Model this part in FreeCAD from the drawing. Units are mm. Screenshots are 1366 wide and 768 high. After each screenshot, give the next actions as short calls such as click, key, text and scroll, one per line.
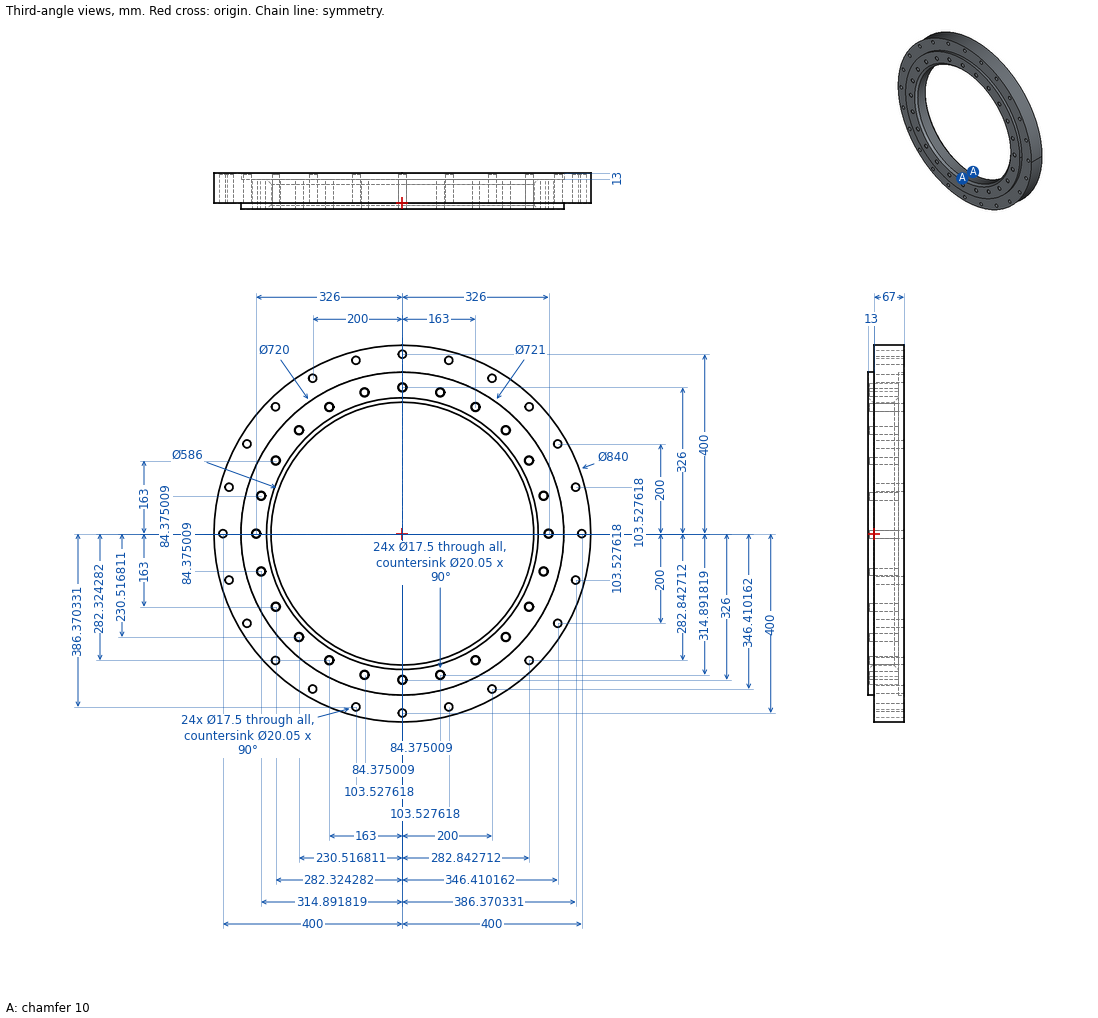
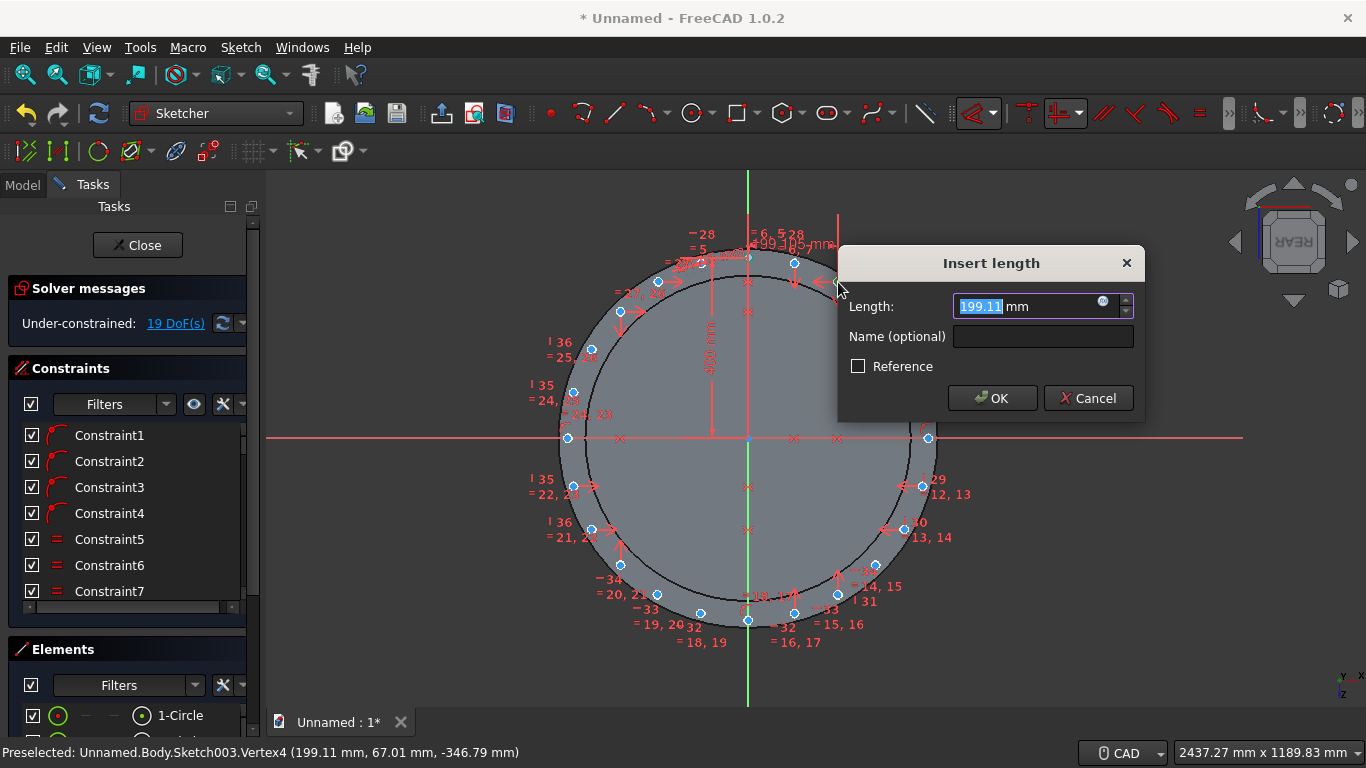
text(200)
key(Return)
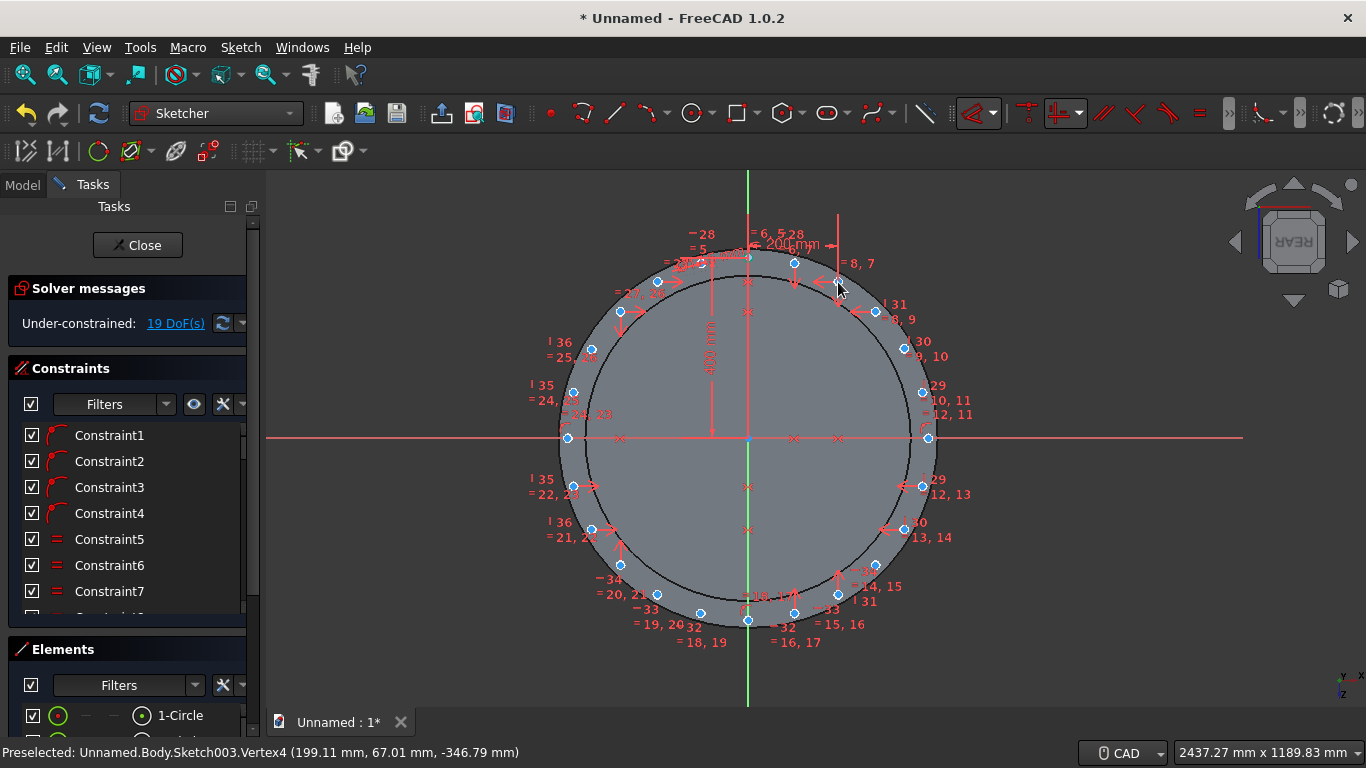
click(904, 349)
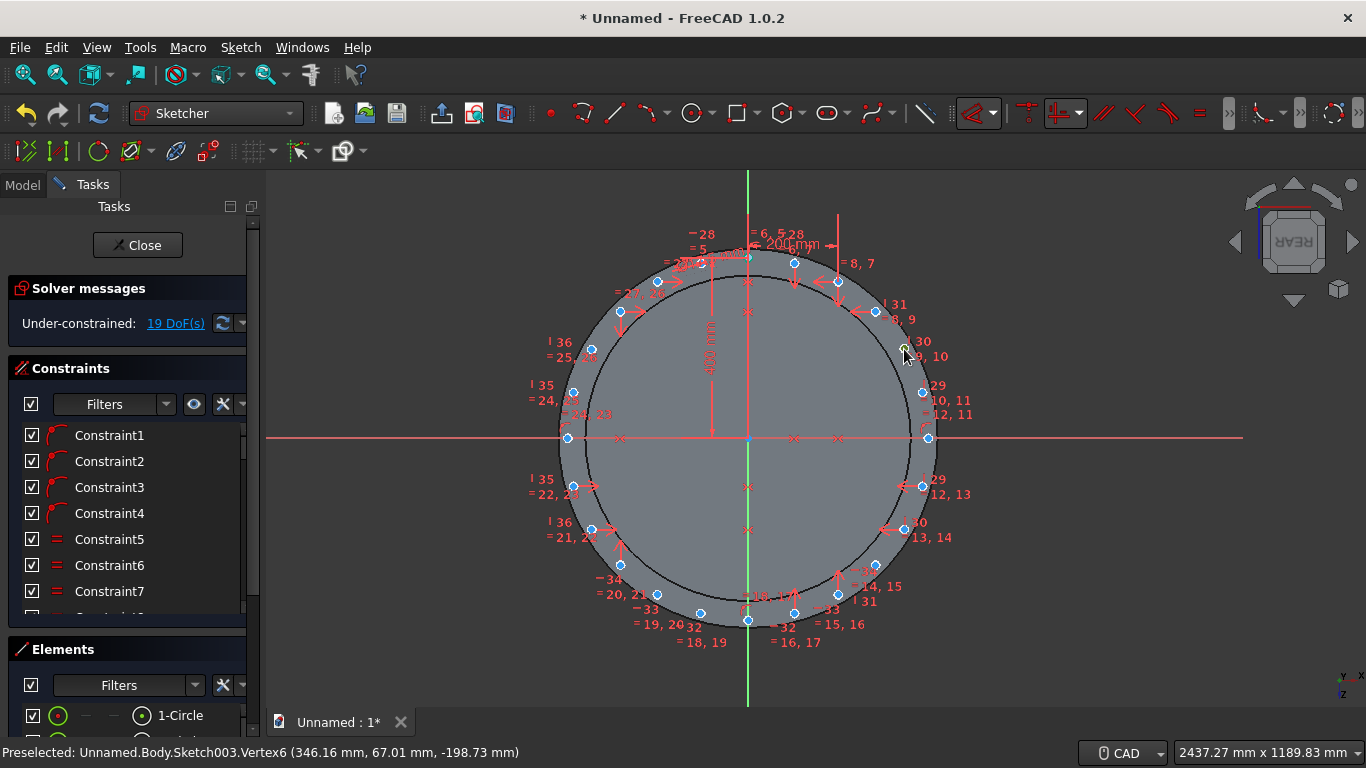
key(i)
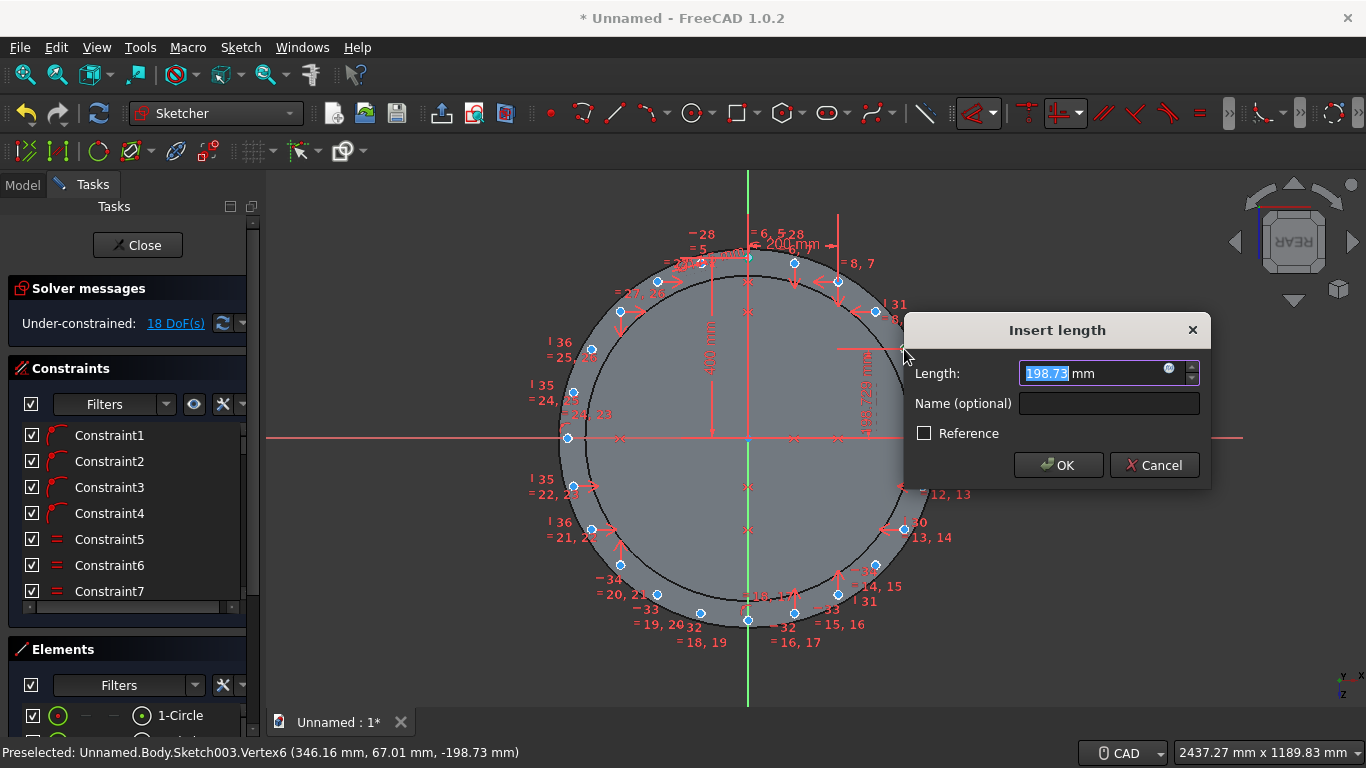
text(200)
key(Return)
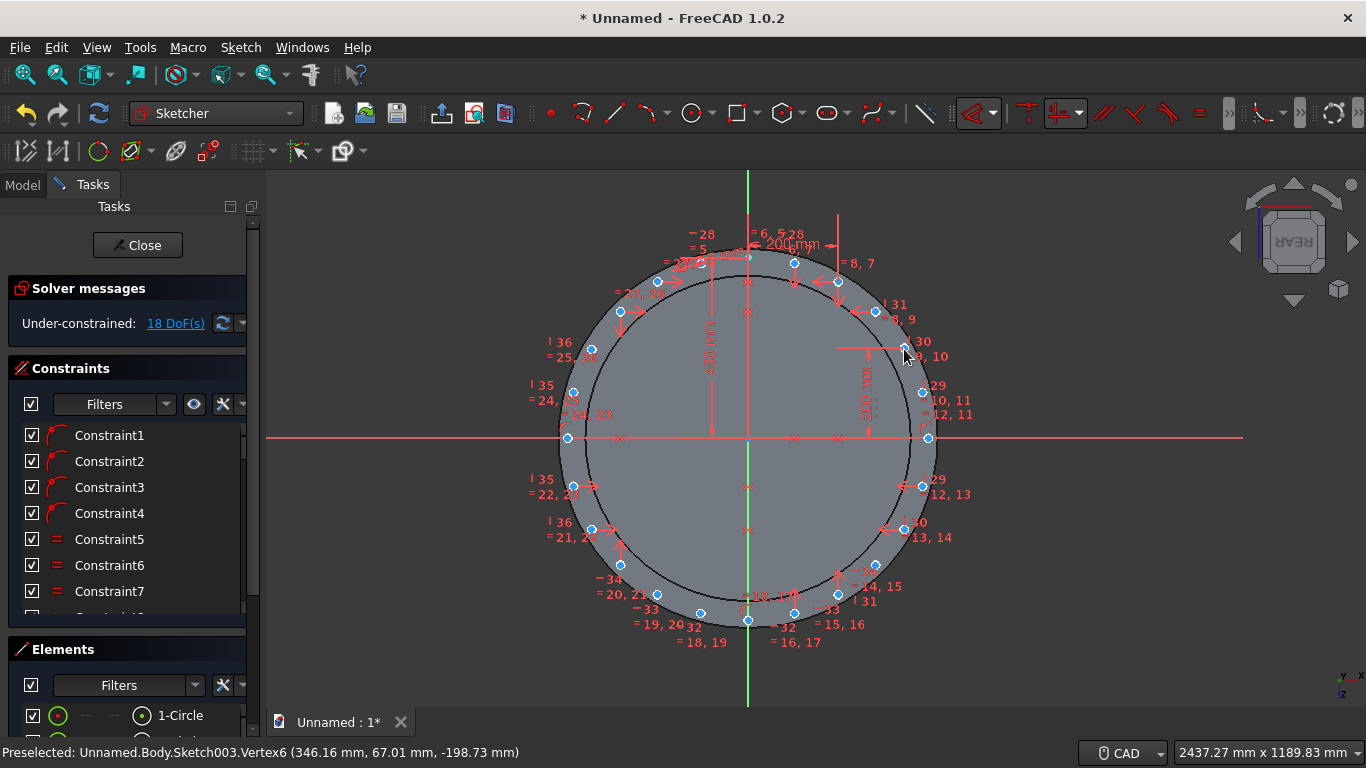
click(928, 438)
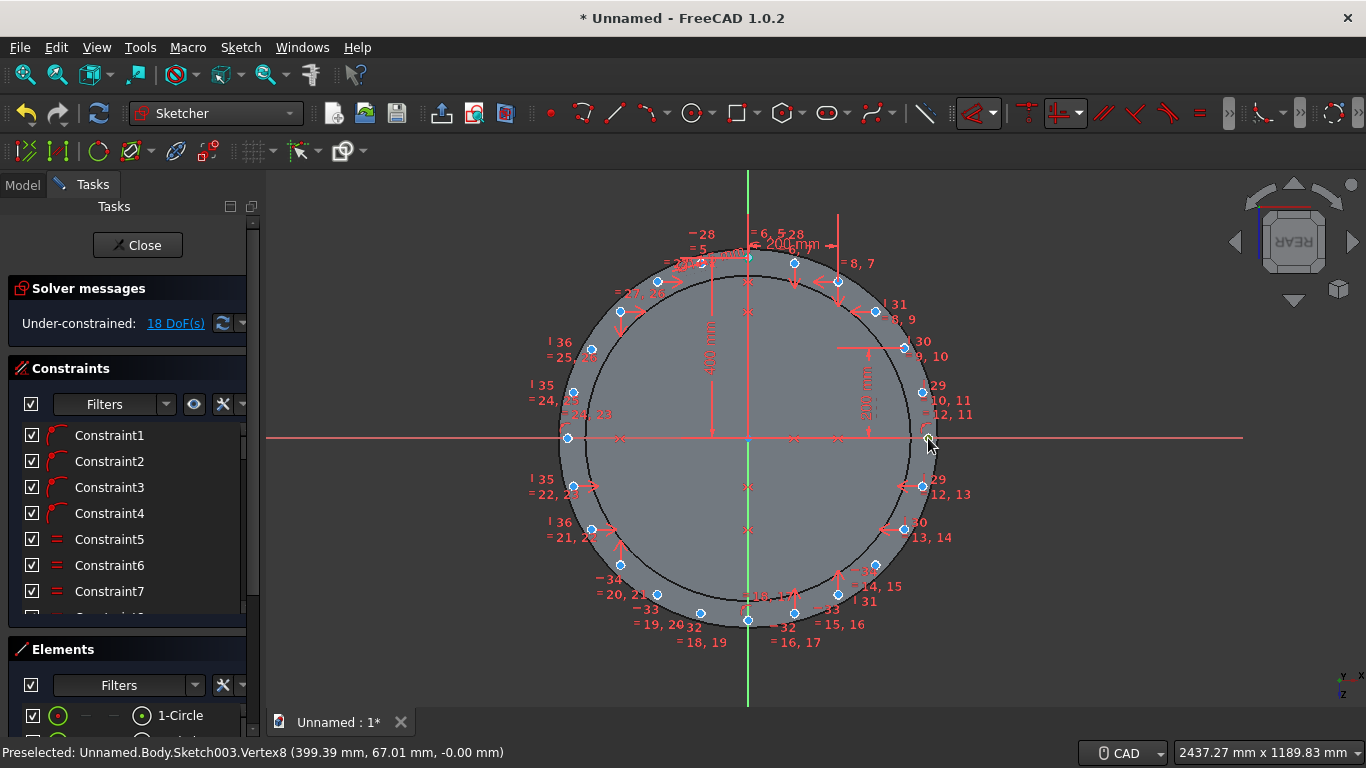
key(l)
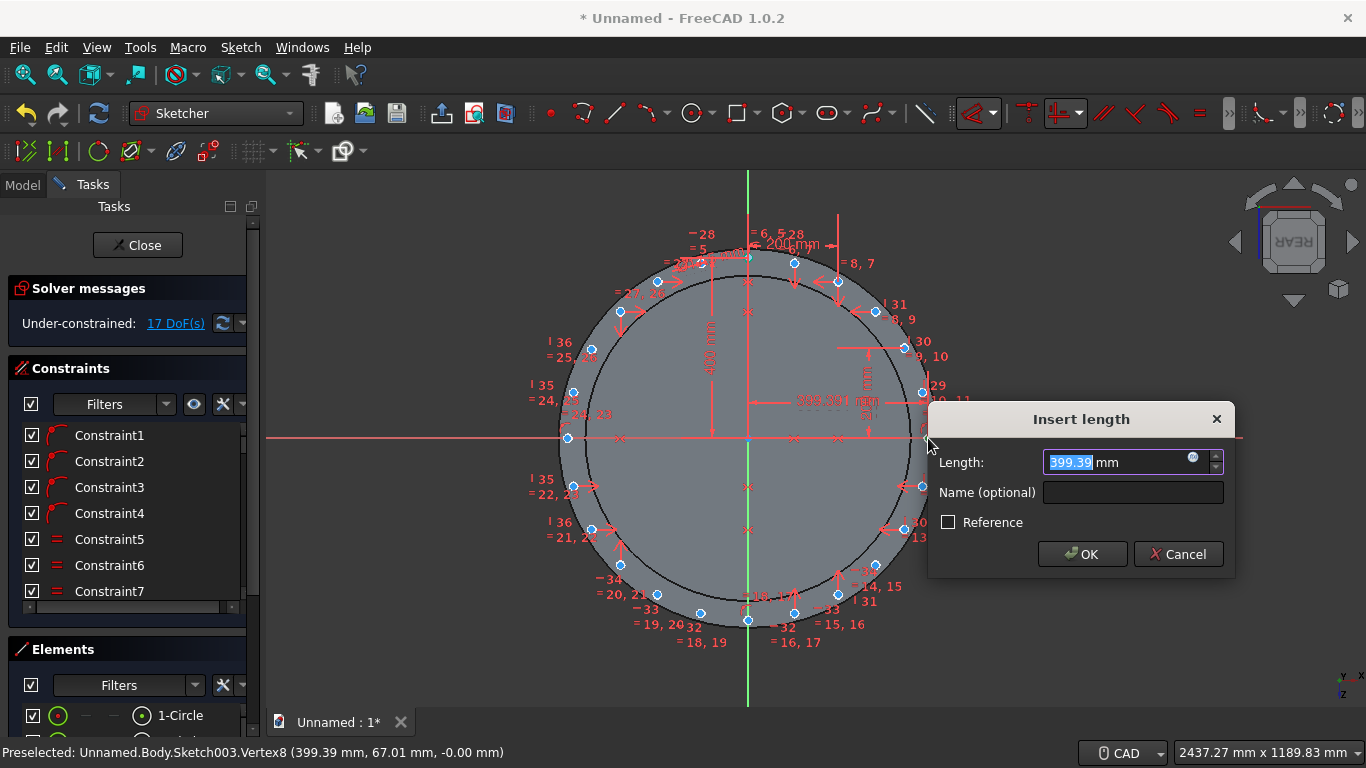
text(400)
key(Return)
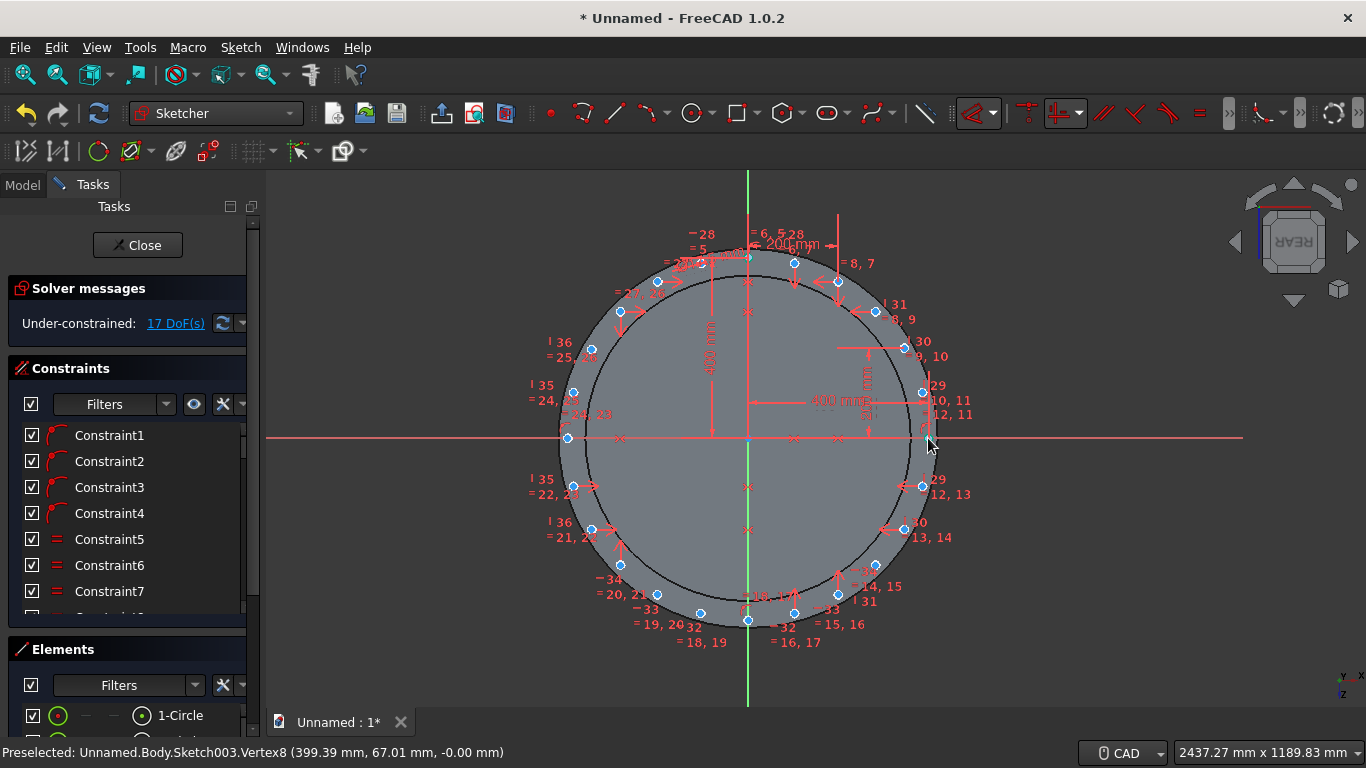
scroll(904, 530, up, 4)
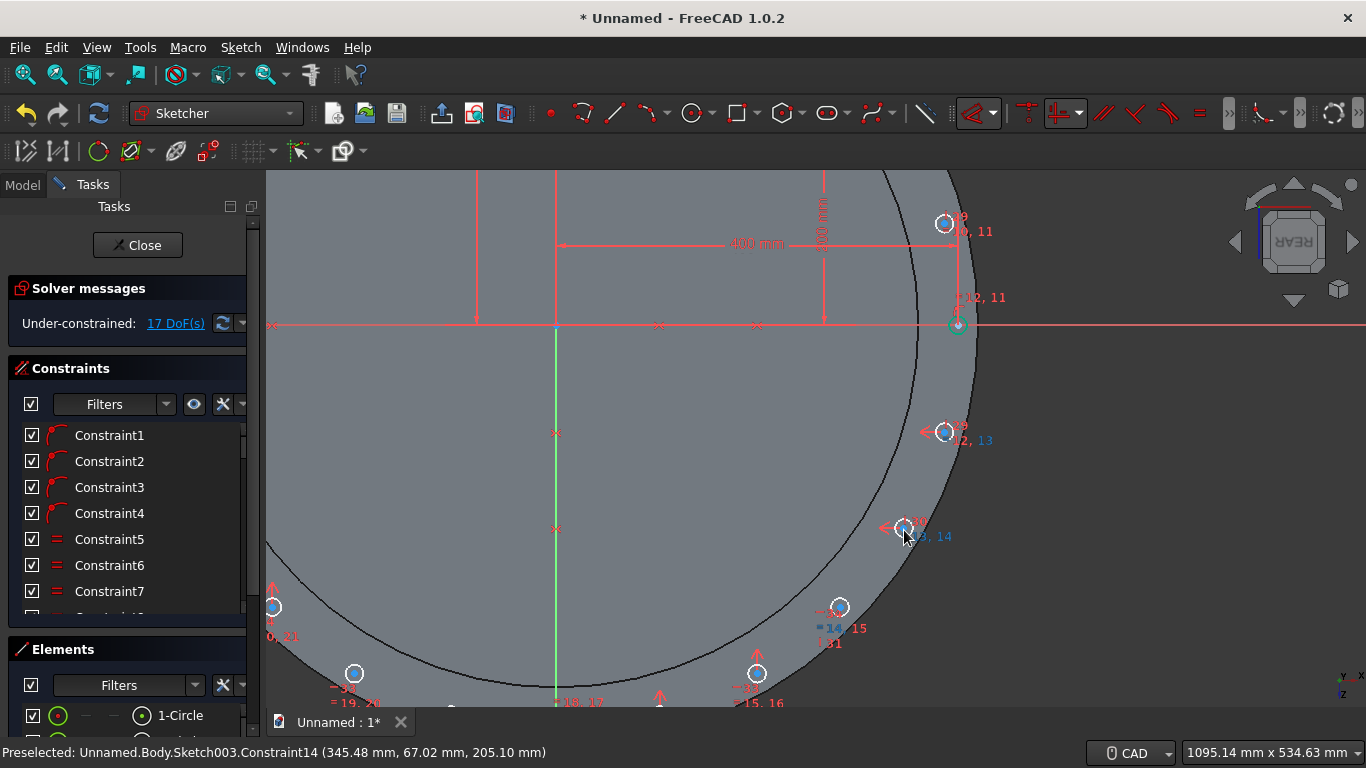
scroll(904, 528, up, 4)